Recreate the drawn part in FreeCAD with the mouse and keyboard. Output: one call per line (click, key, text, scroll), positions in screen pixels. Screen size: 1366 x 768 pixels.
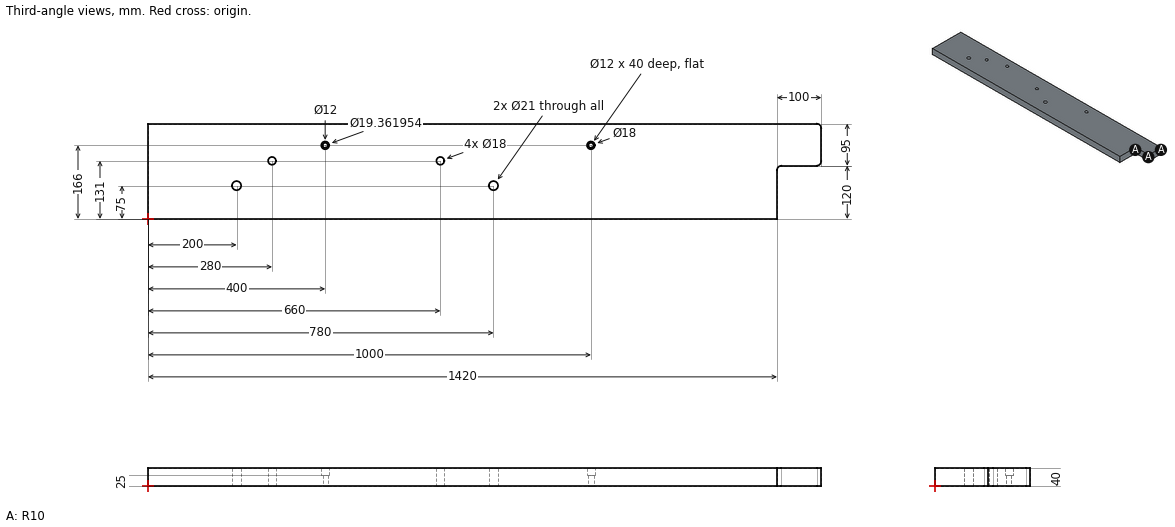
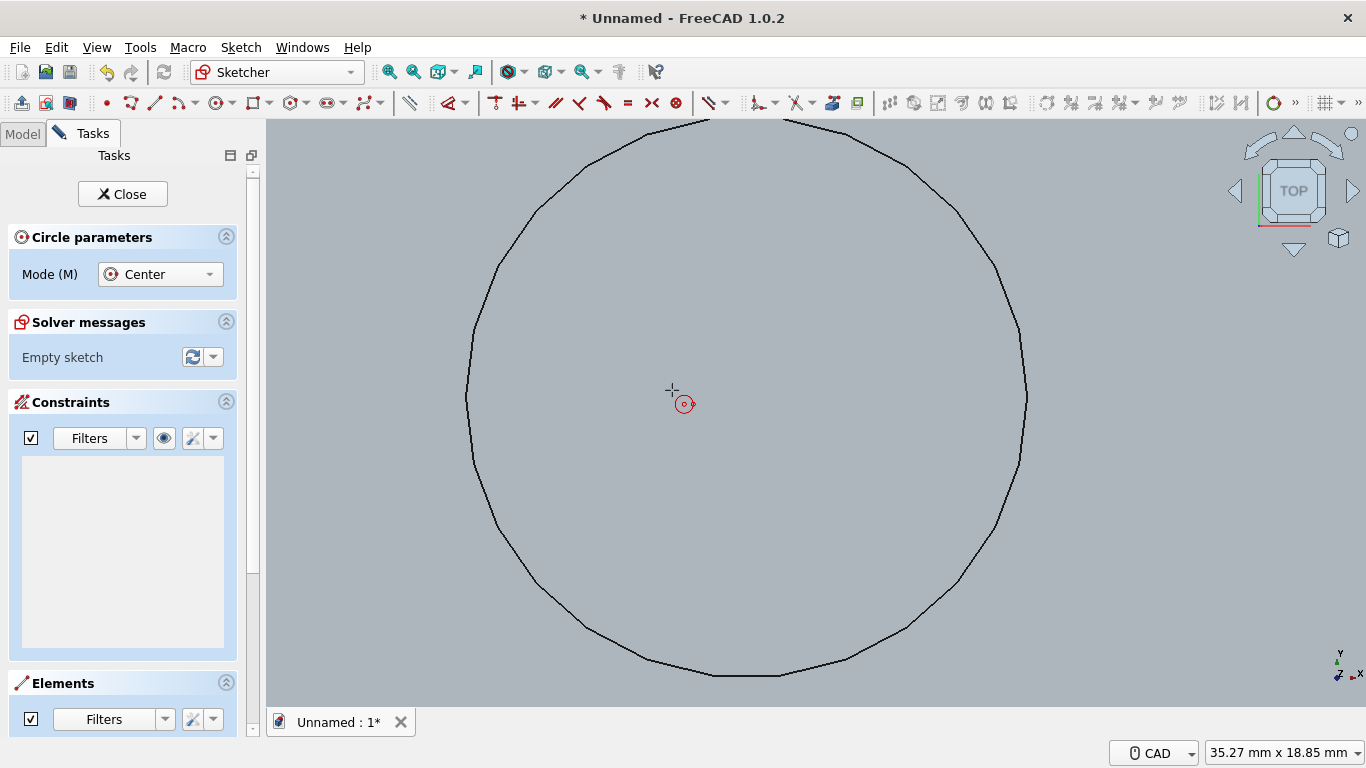
click(747, 397)
click(879, 265)
key(Escape)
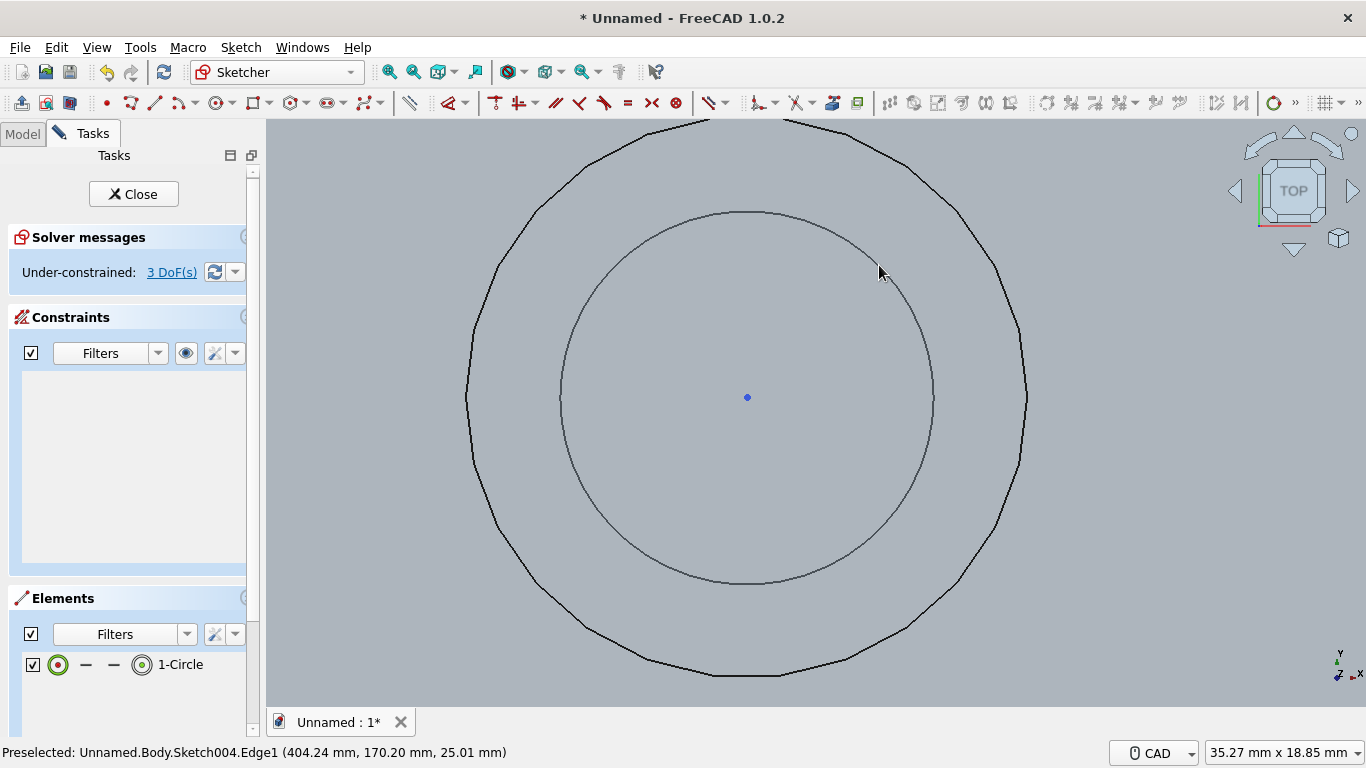
key(d)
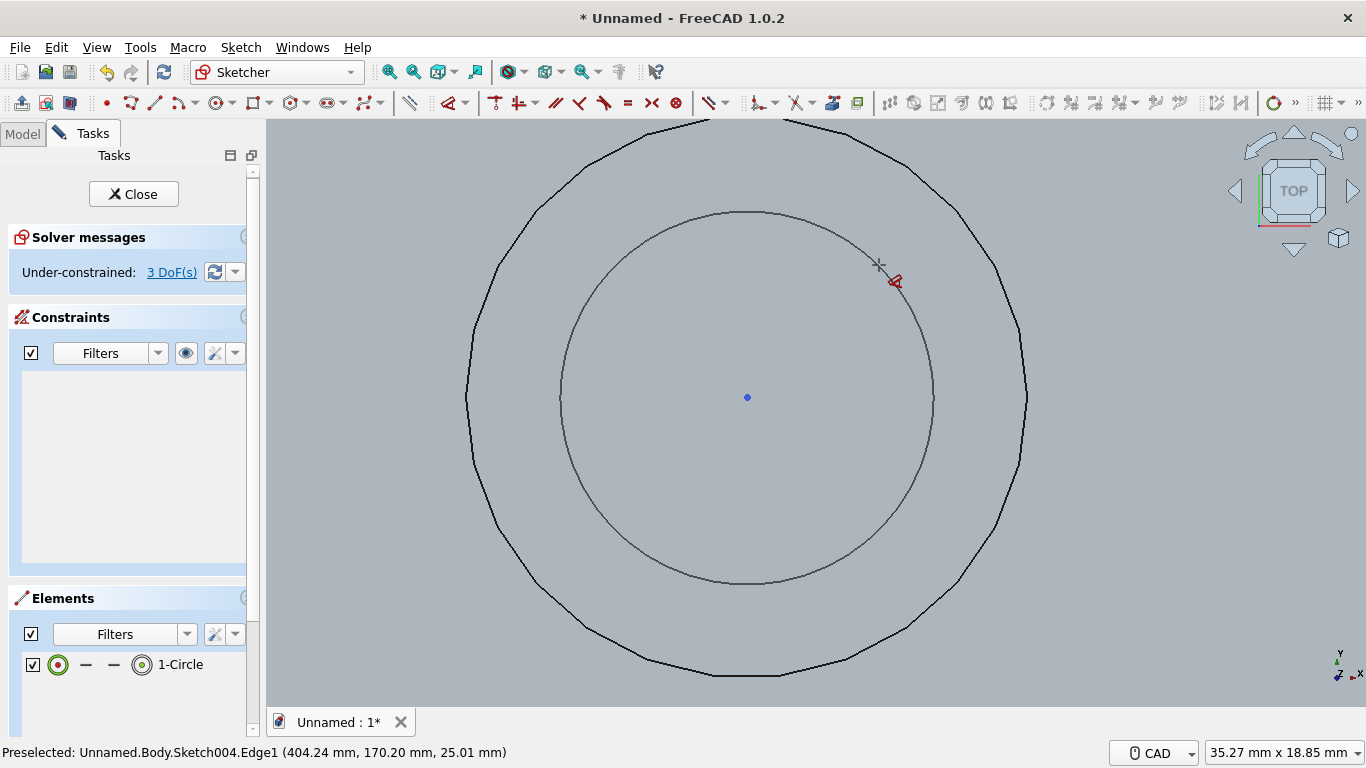
click(879, 266)
click(902, 243)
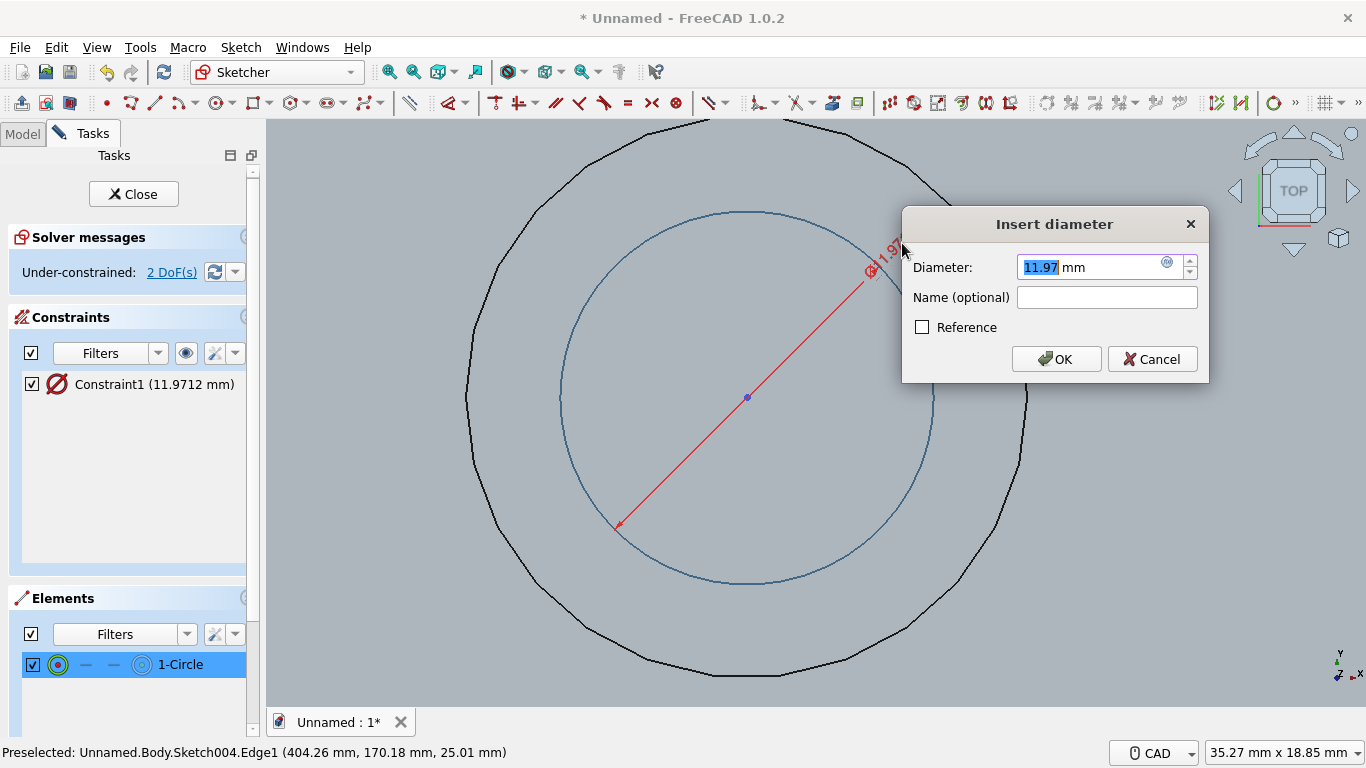
text(12)
key(Return)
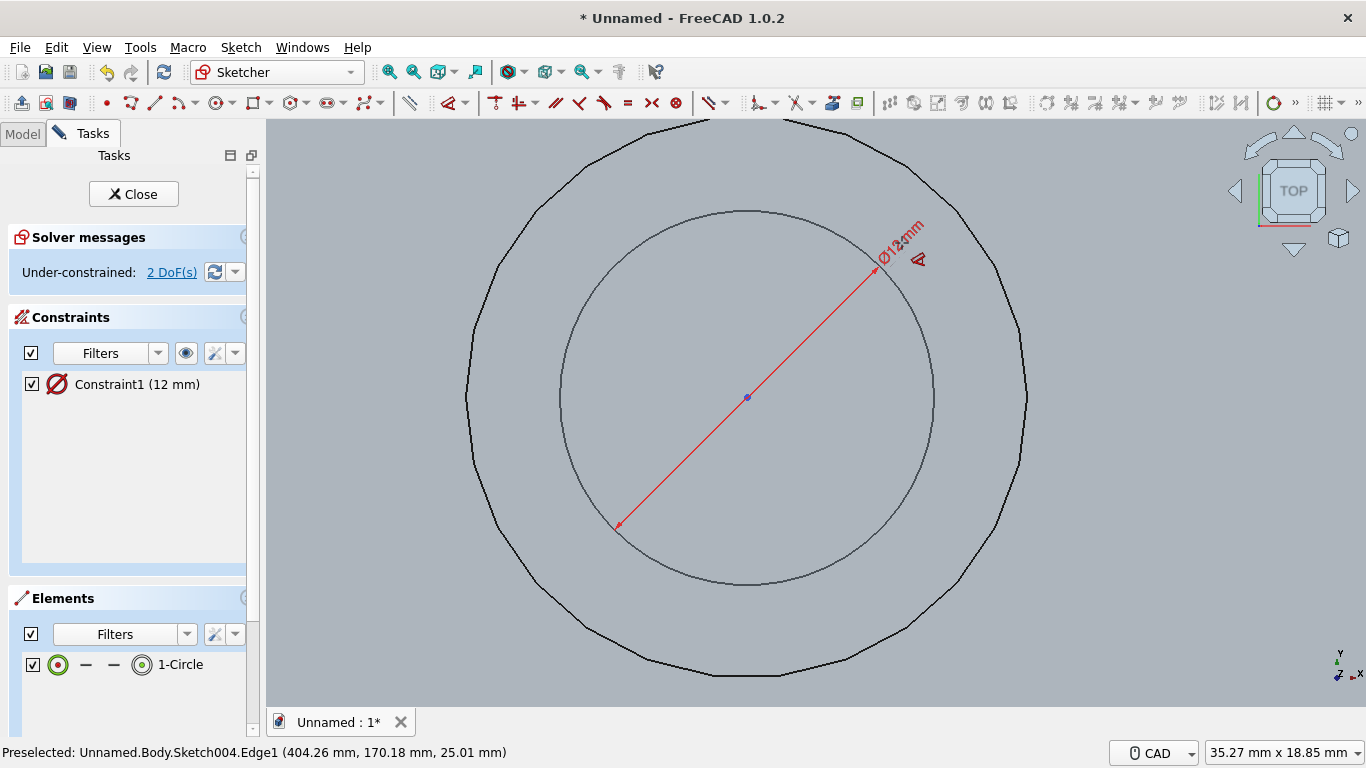
click(747, 398)
click(520, 364)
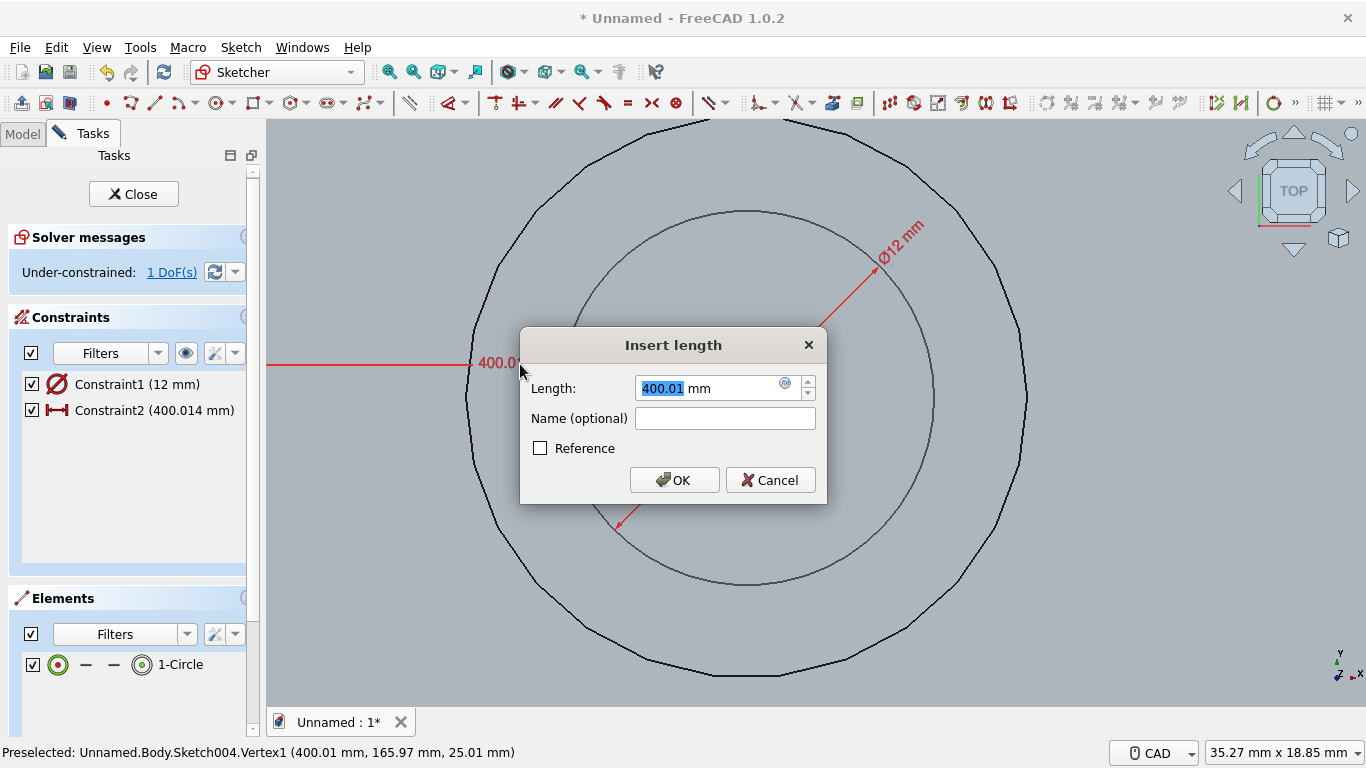
text(400)
key(Return)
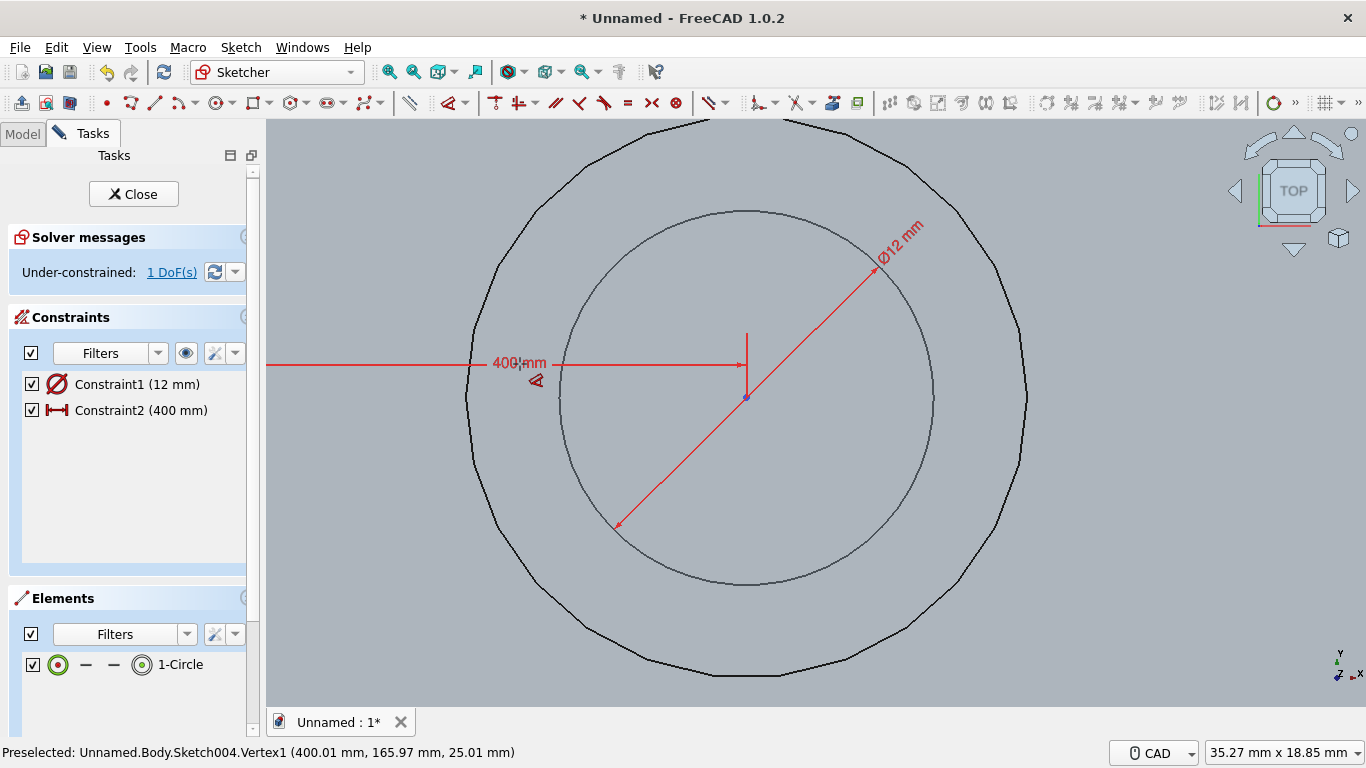
click(747, 398)
click(781, 539)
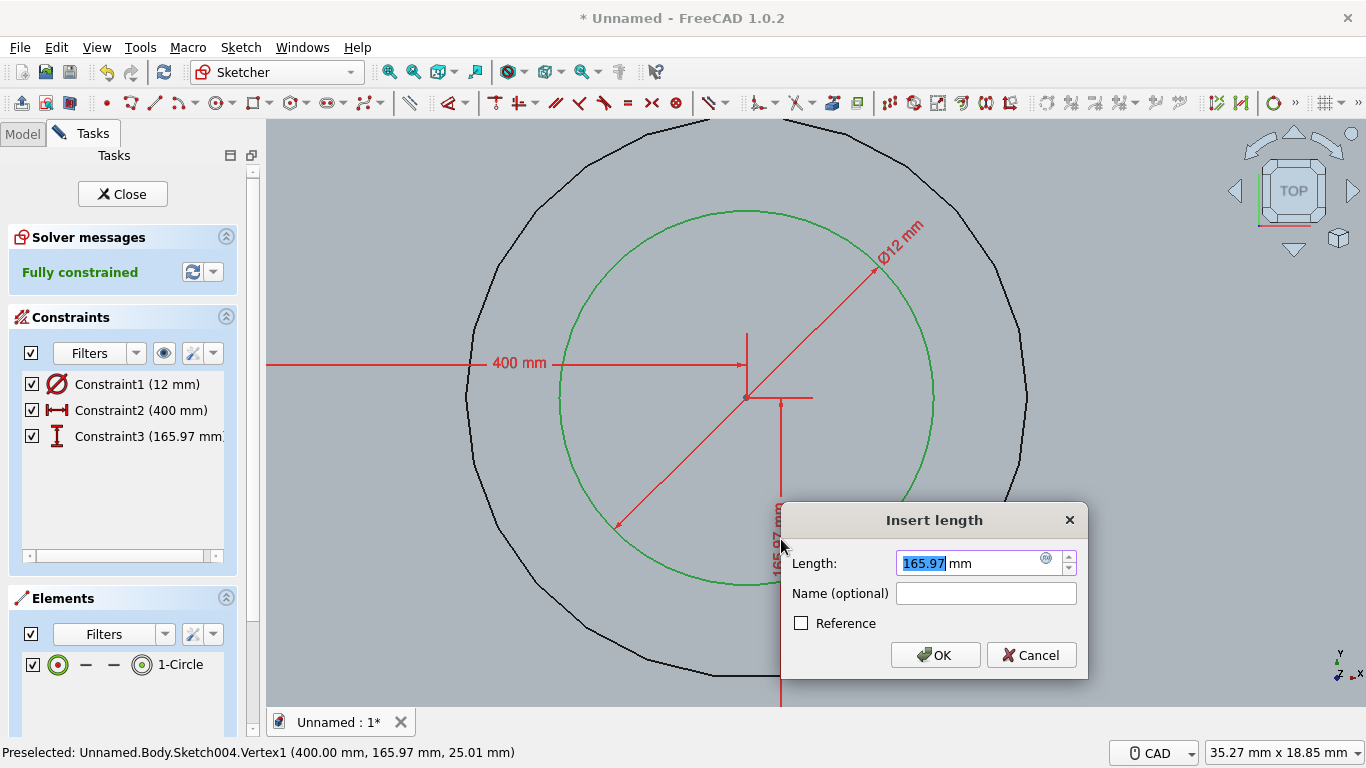
text(166)
key(Return)
key(Escape)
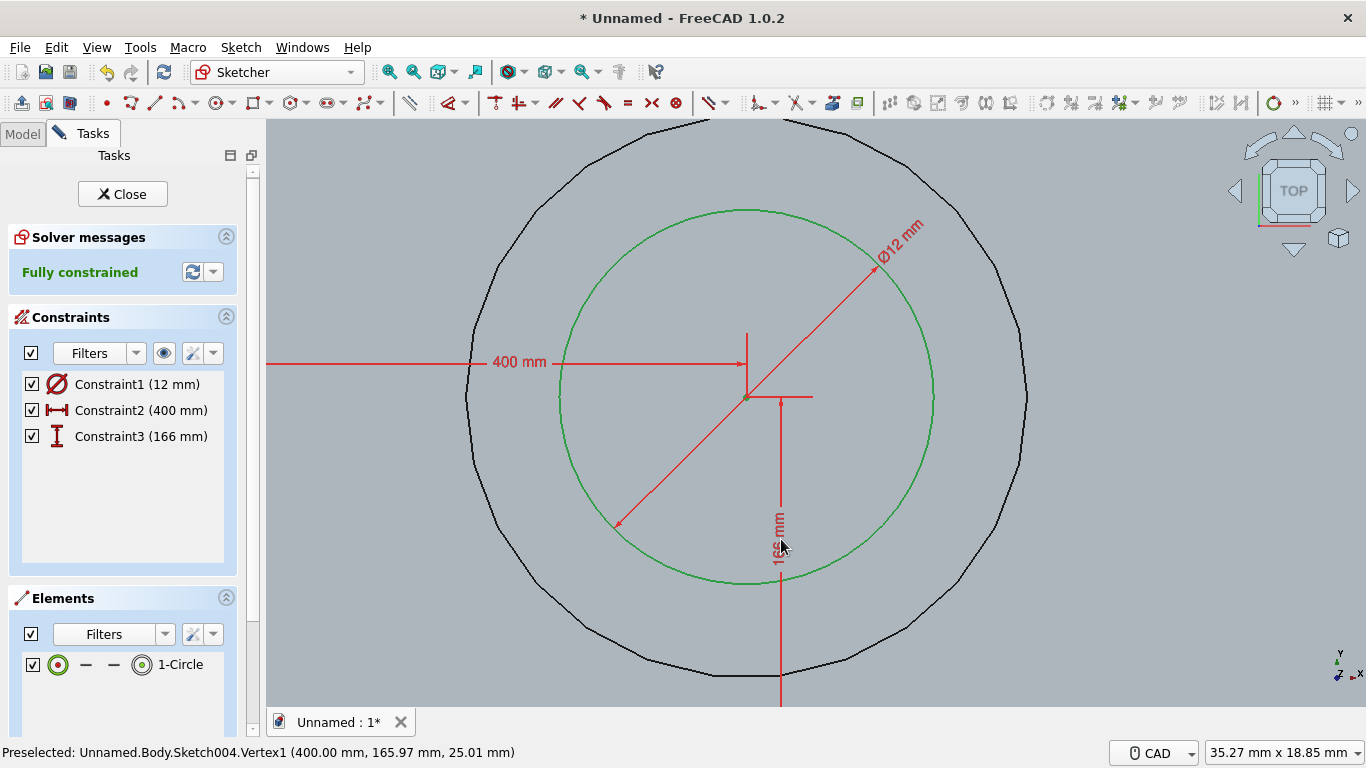
click(123, 194)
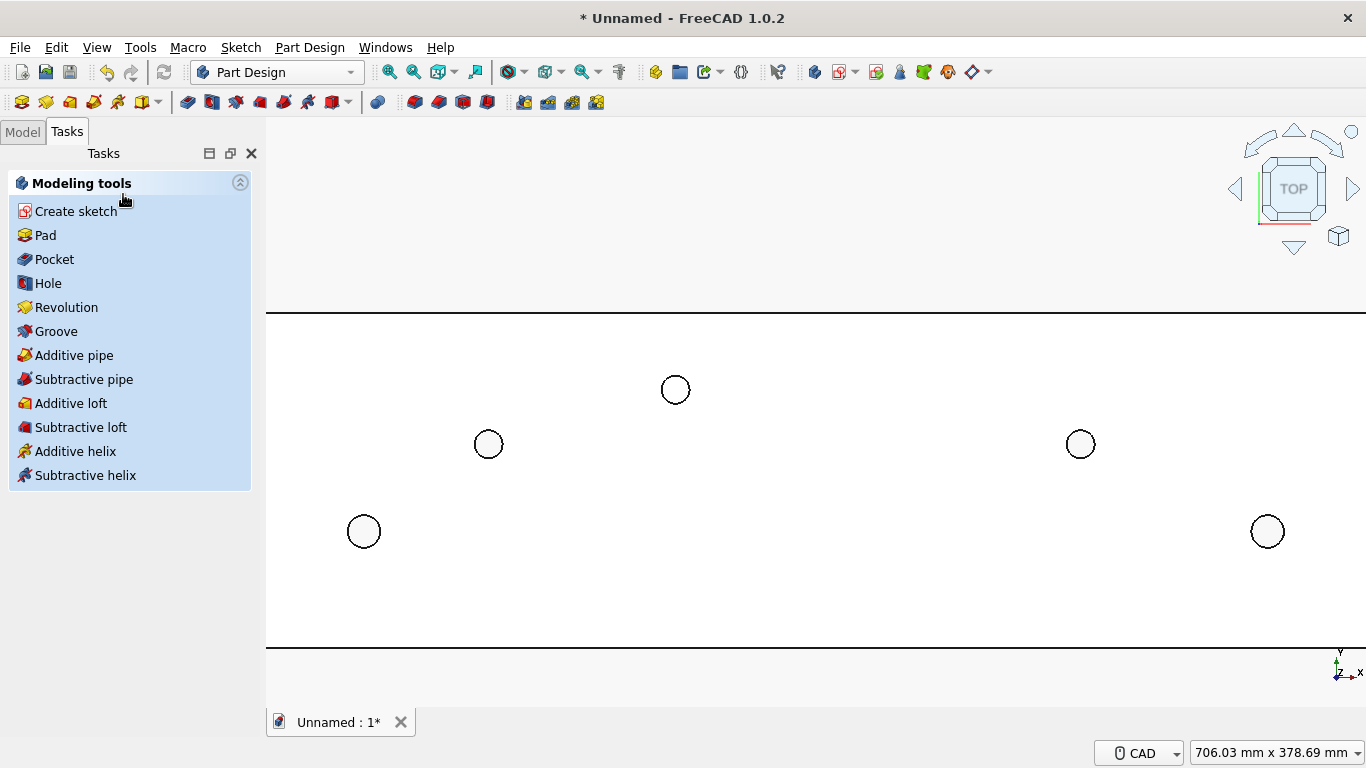
click(188, 102)